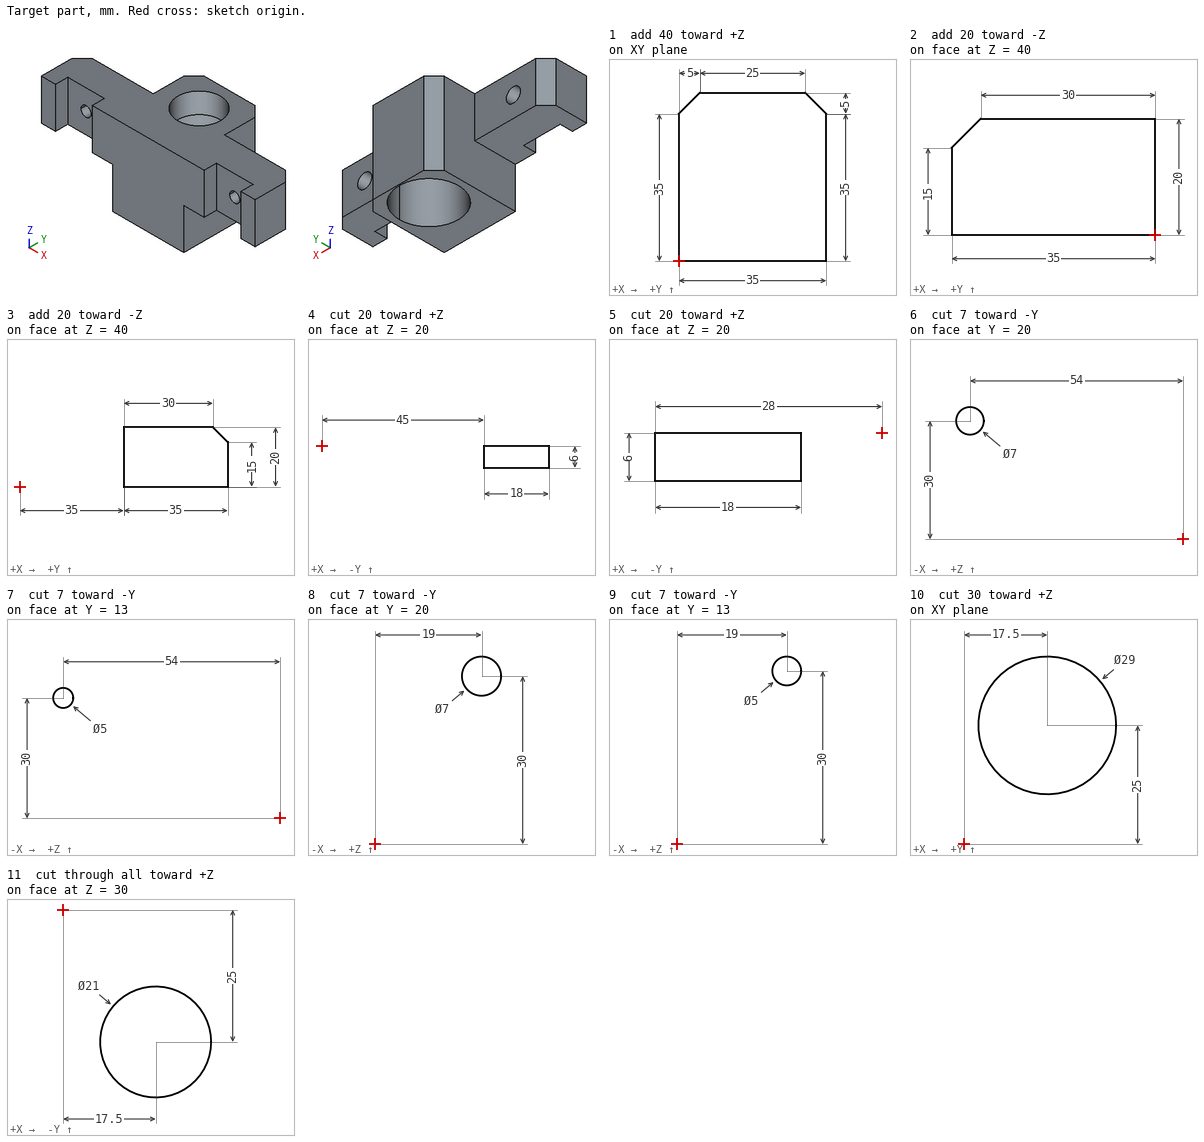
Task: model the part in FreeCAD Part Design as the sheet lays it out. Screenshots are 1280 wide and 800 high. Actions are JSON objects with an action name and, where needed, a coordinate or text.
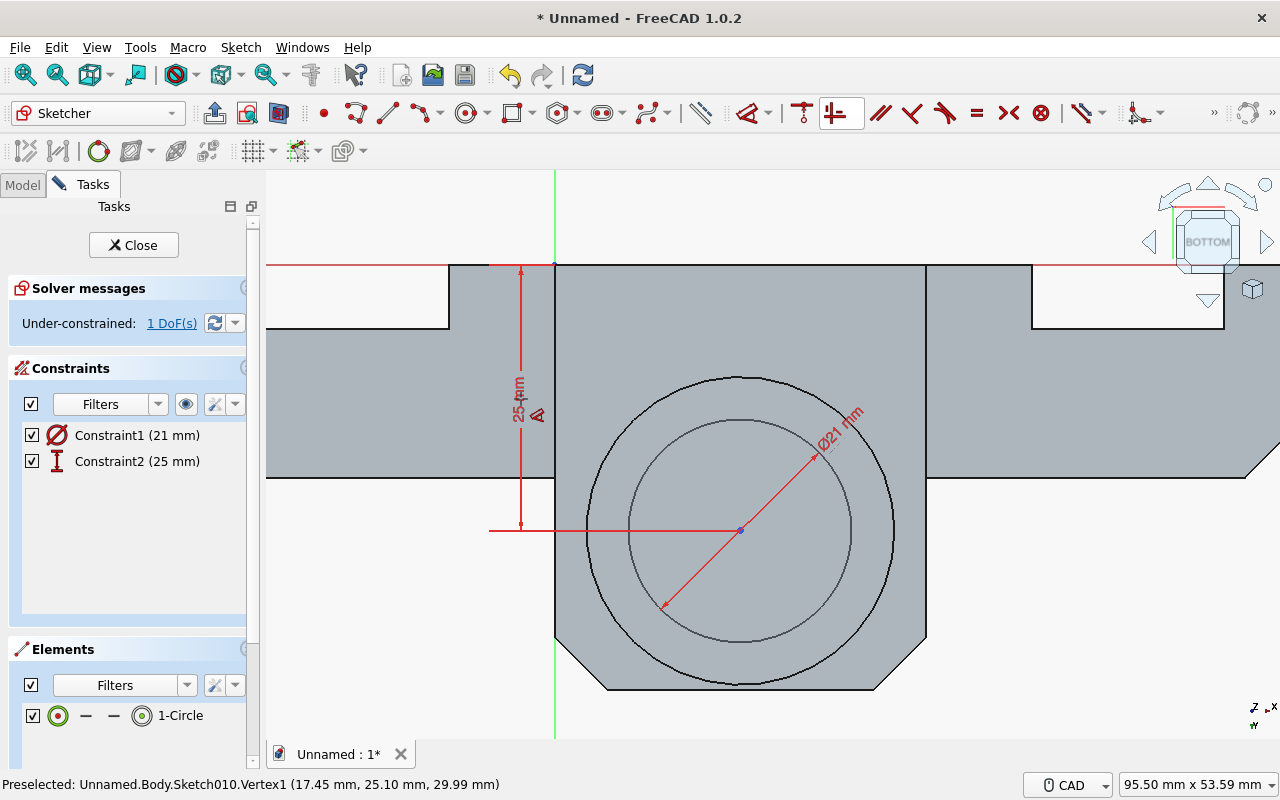
{"action": "left_click", "coordinate": [740, 531]}
{"action": "left_click", "coordinate": [647, 231]}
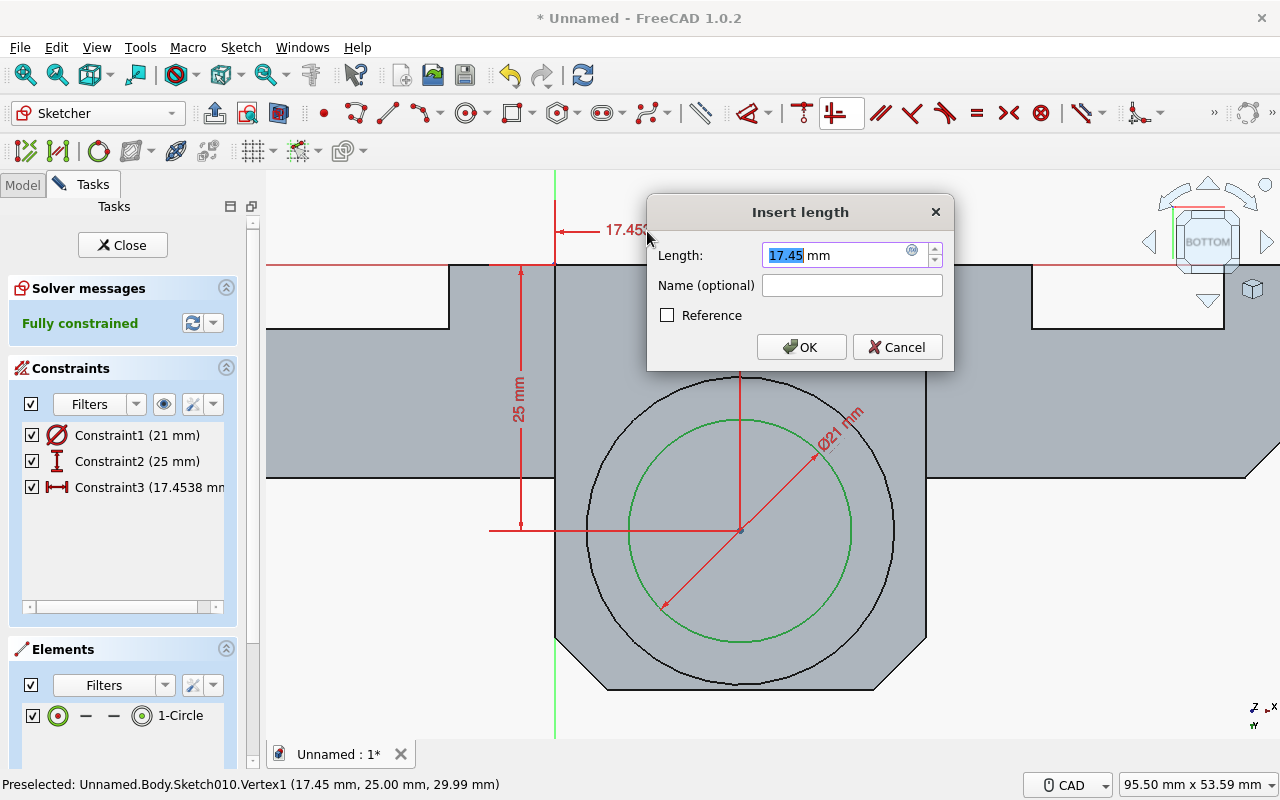
{"action": "type", "text": "17.5"}
{"action": "key", "text": "Return"}
{"action": "key", "text": "Escape"}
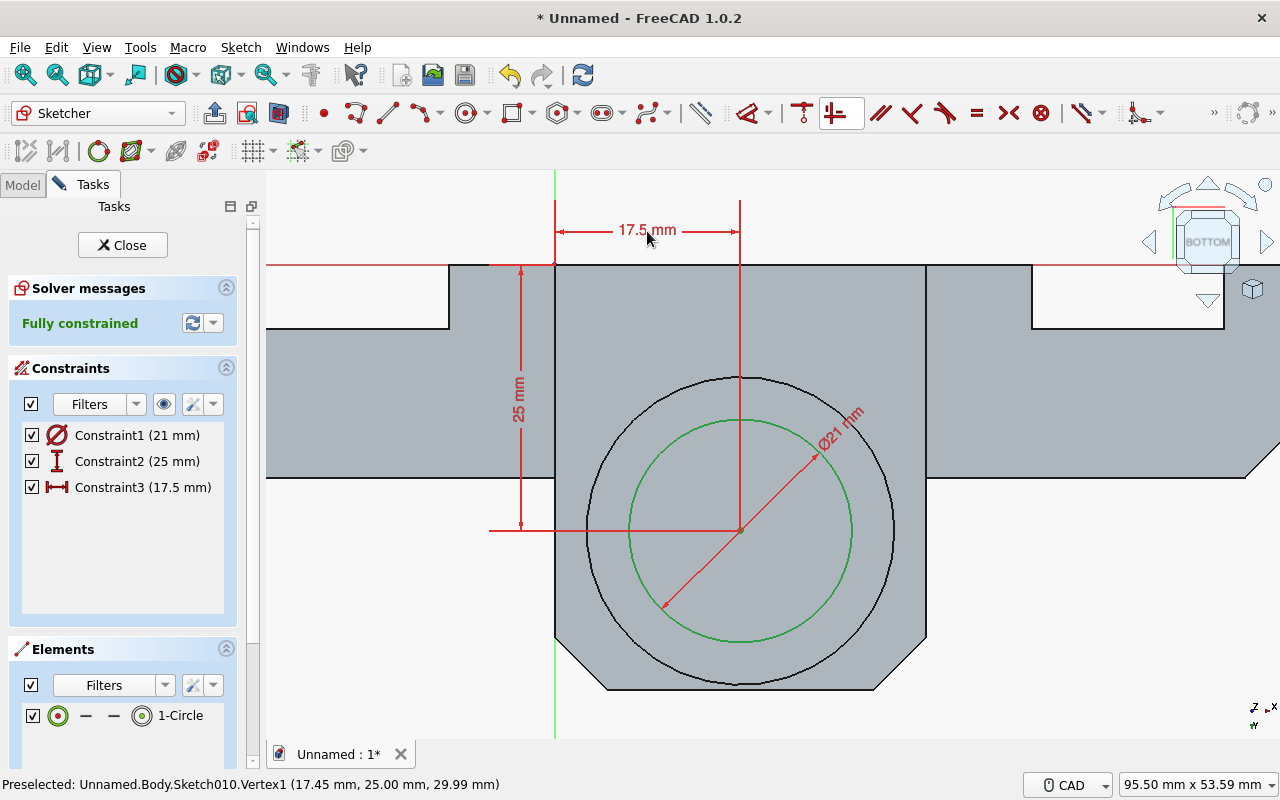
{"action": "left_click", "coordinate": [123, 245]}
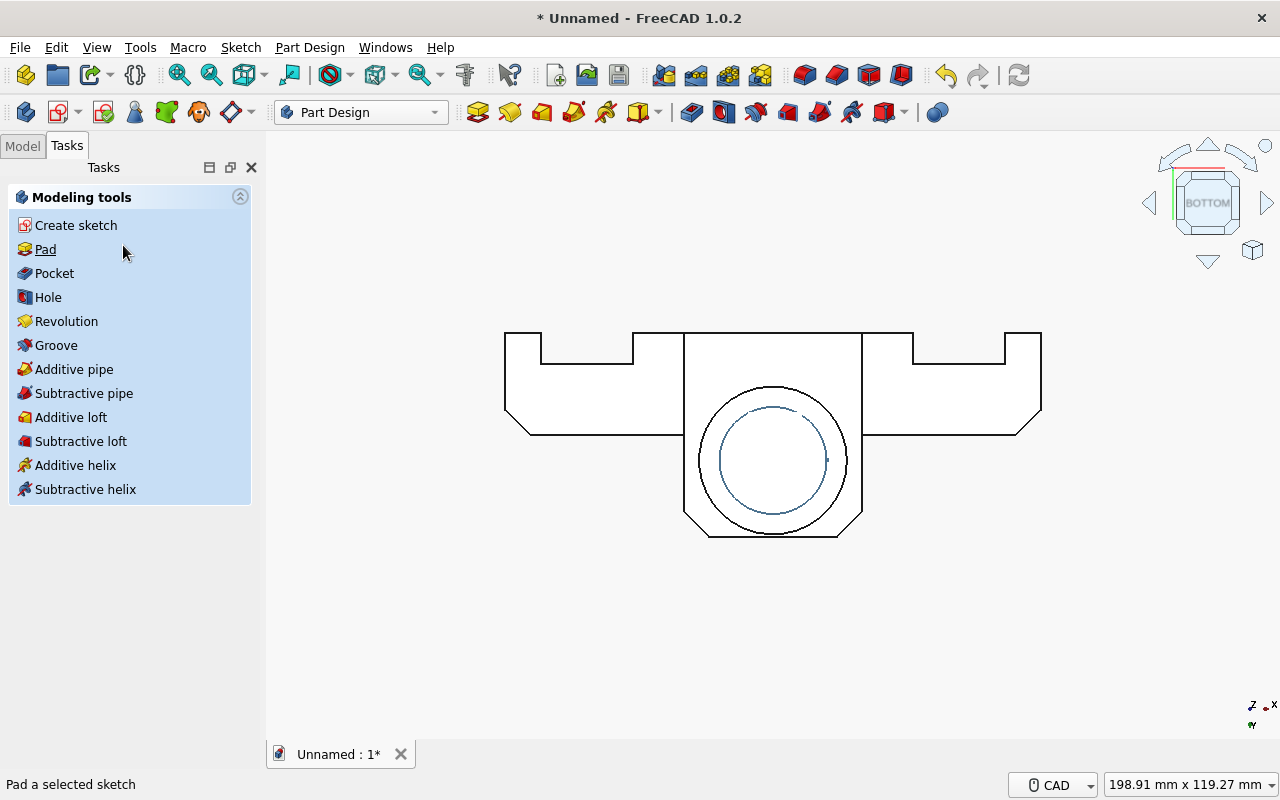
{"action": "left_click", "coordinate": [692, 112]}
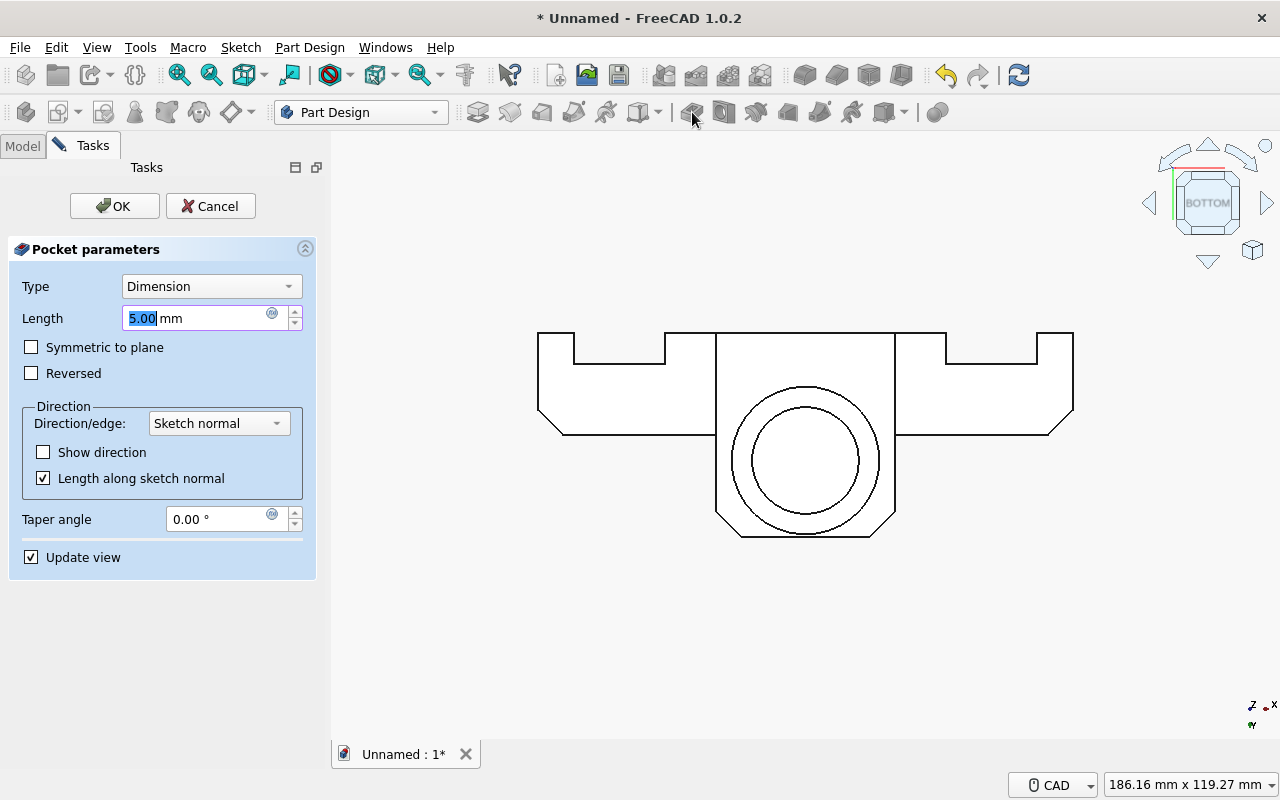
{"action": "left_click", "coordinate": [212, 286]}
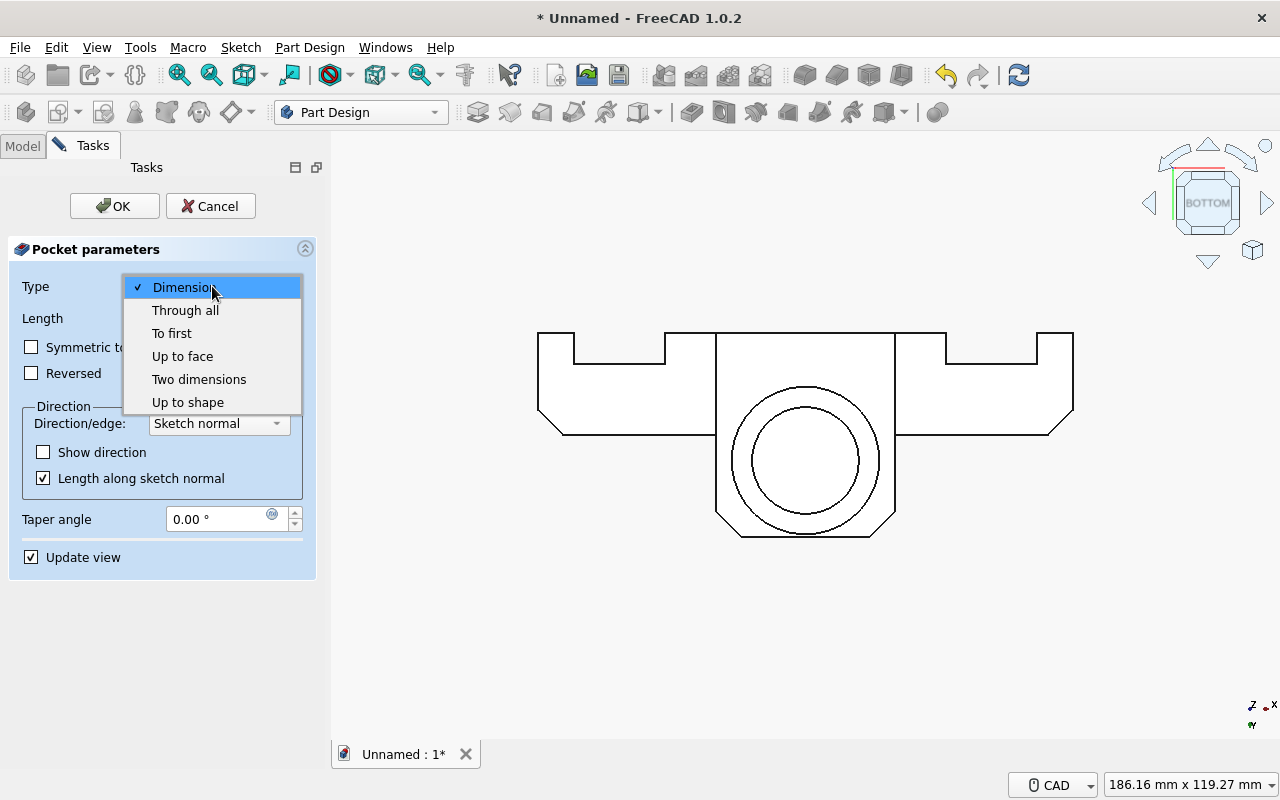
{"action": "left_click", "coordinate": [212, 310]}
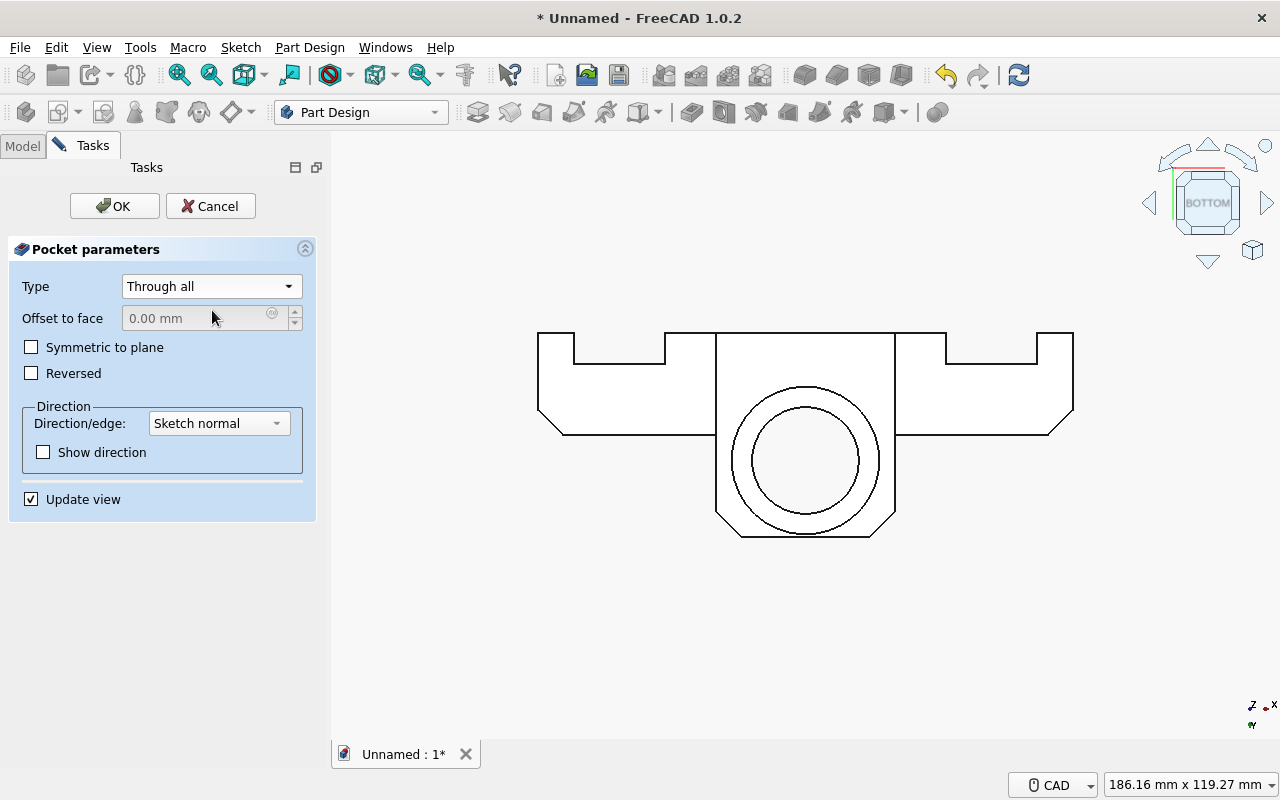
{"action": "left_click", "coordinate": [115, 206]}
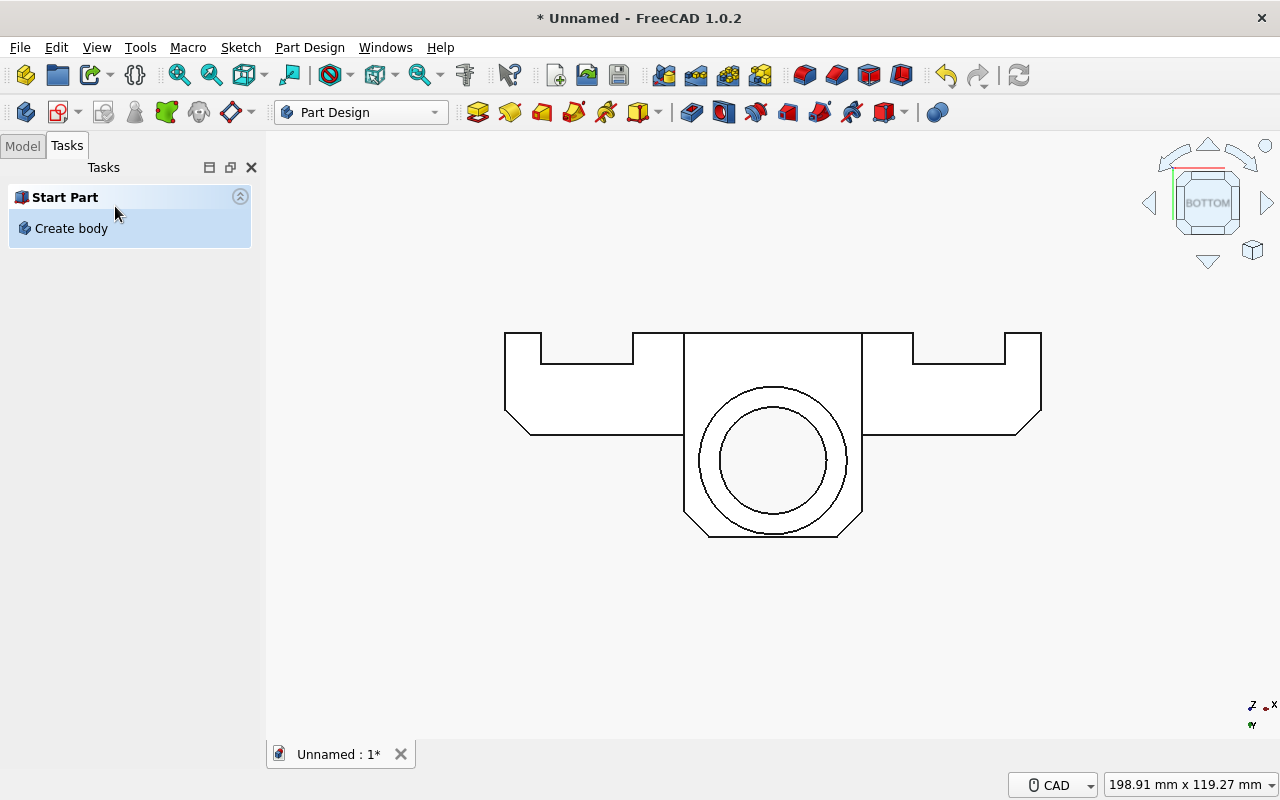
{"action": "key", "text": "0"}